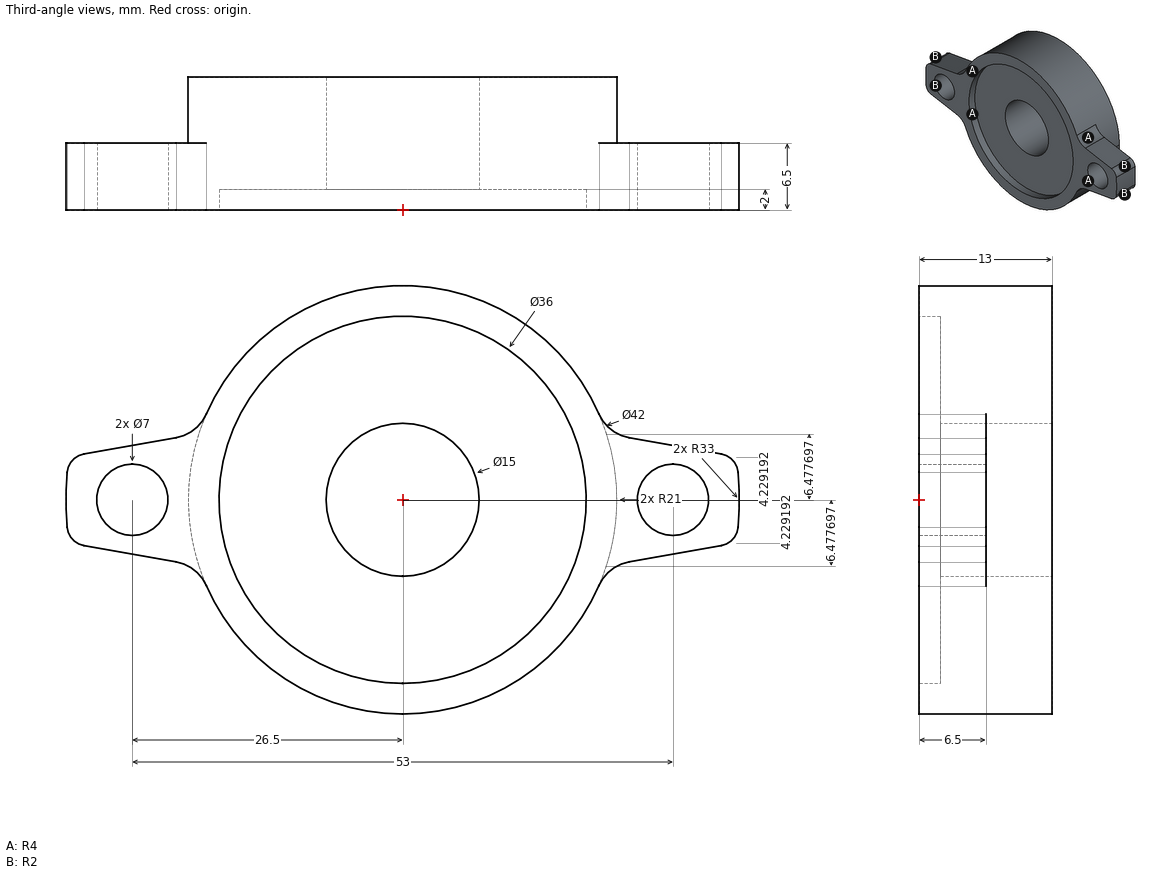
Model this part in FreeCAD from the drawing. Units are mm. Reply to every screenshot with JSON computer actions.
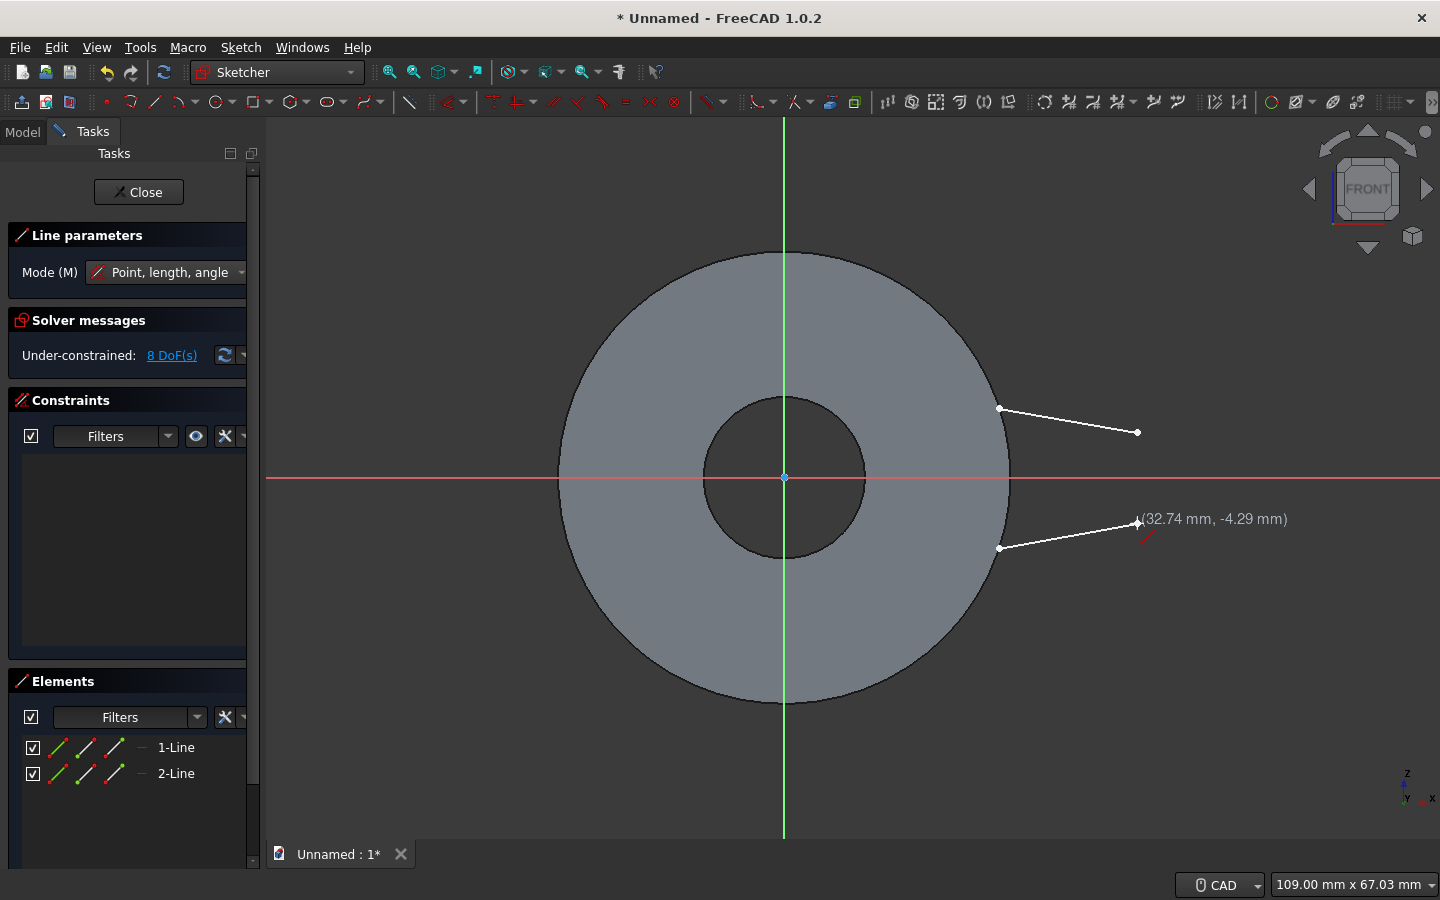
{"action": "key", "text": "g 3 a"}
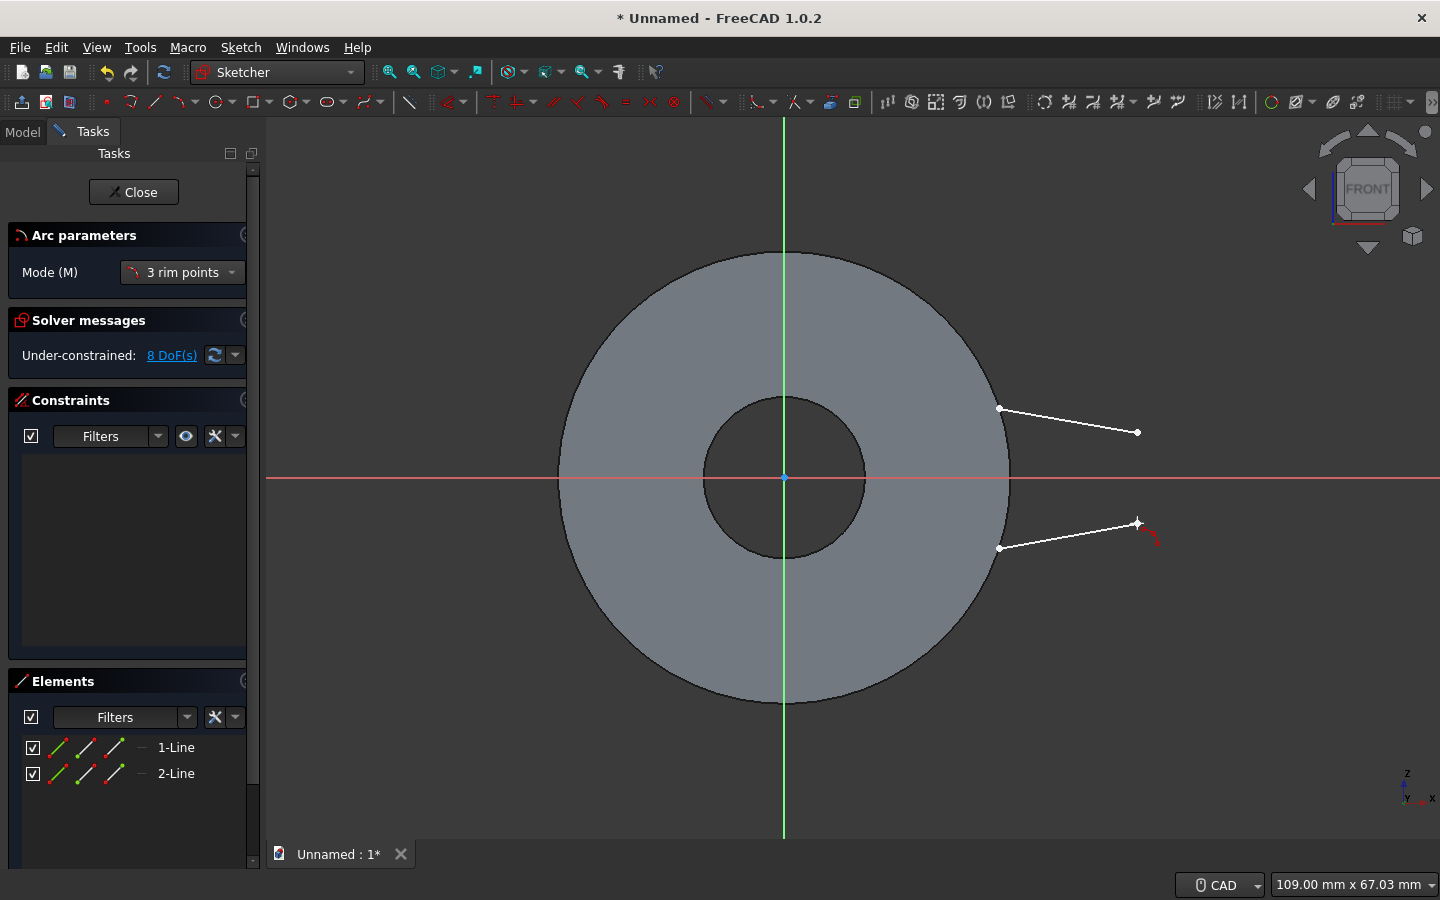
{"action": "left_click", "coordinate": [999, 409]}
{"action": "left_click", "coordinate": [999, 549]}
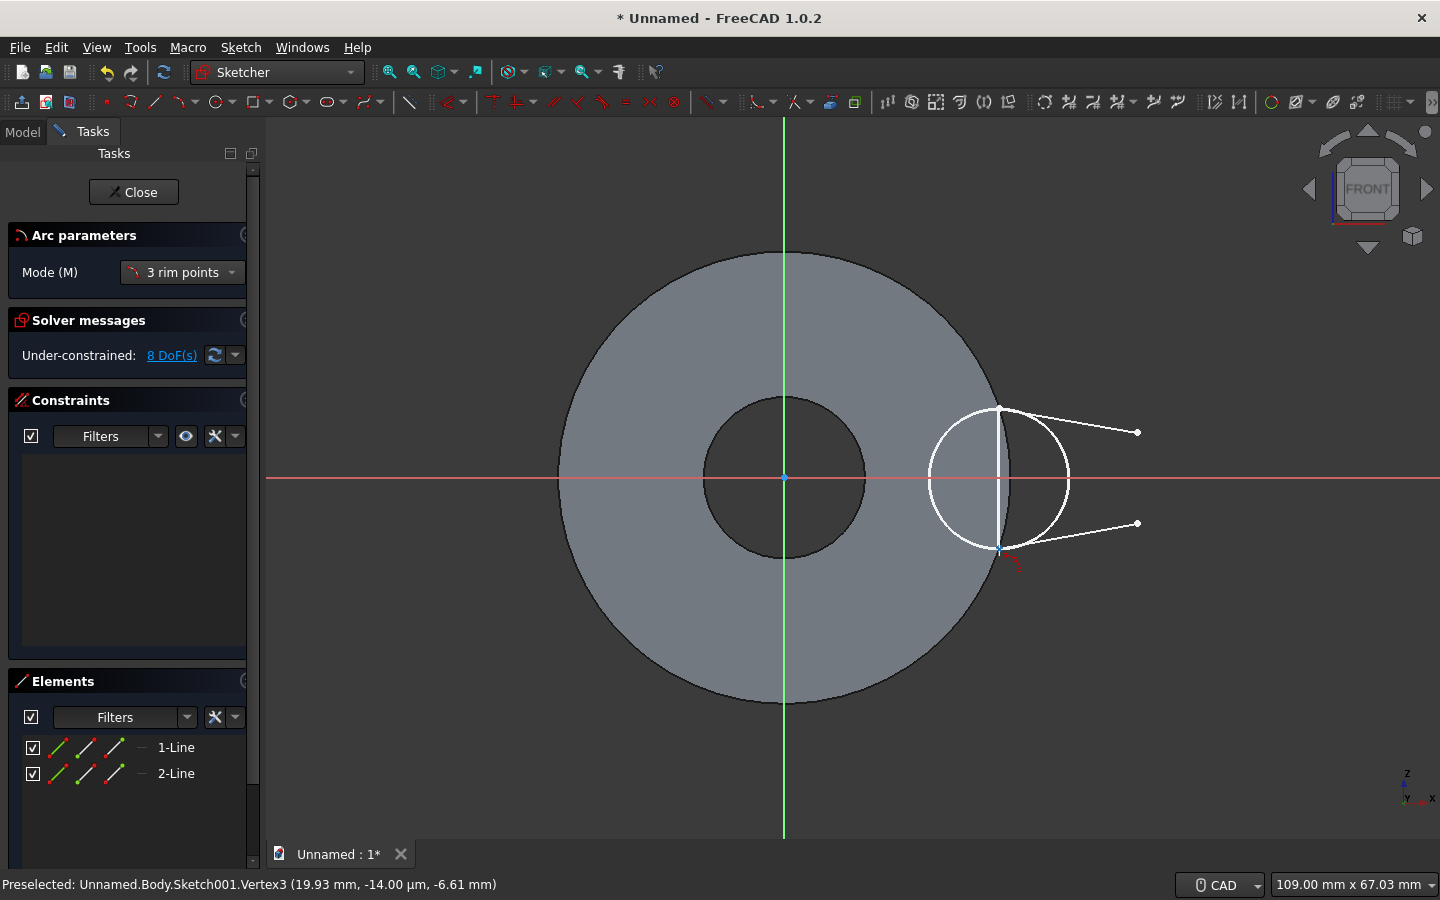
{"action": "scroll", "coordinate": [1010, 492], "scroll_direction": "up", "scroll_amount": 3}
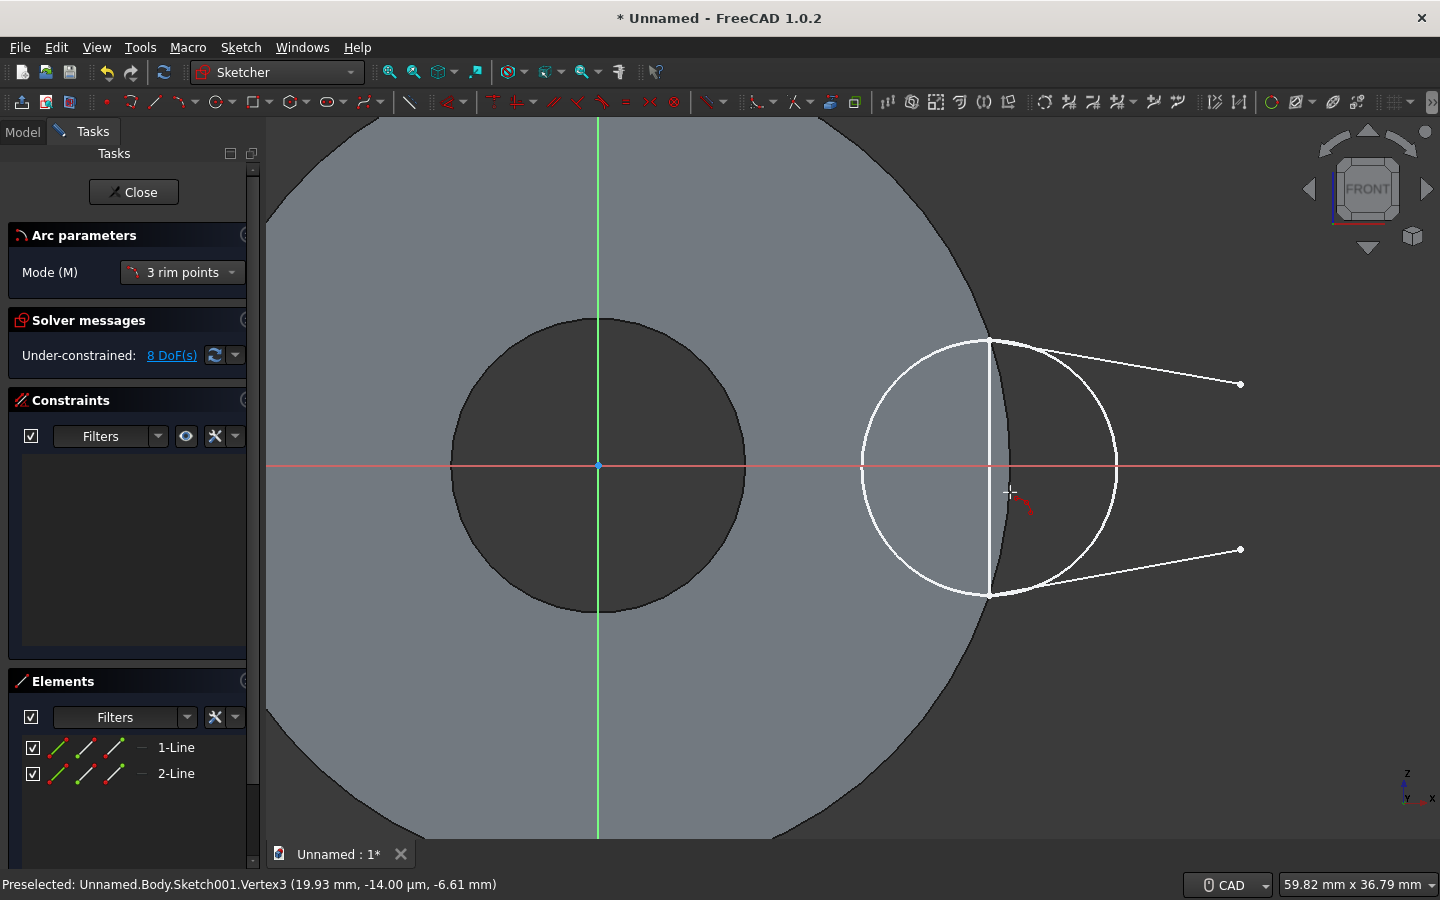
{"action": "left_click", "coordinate": [1010, 491]}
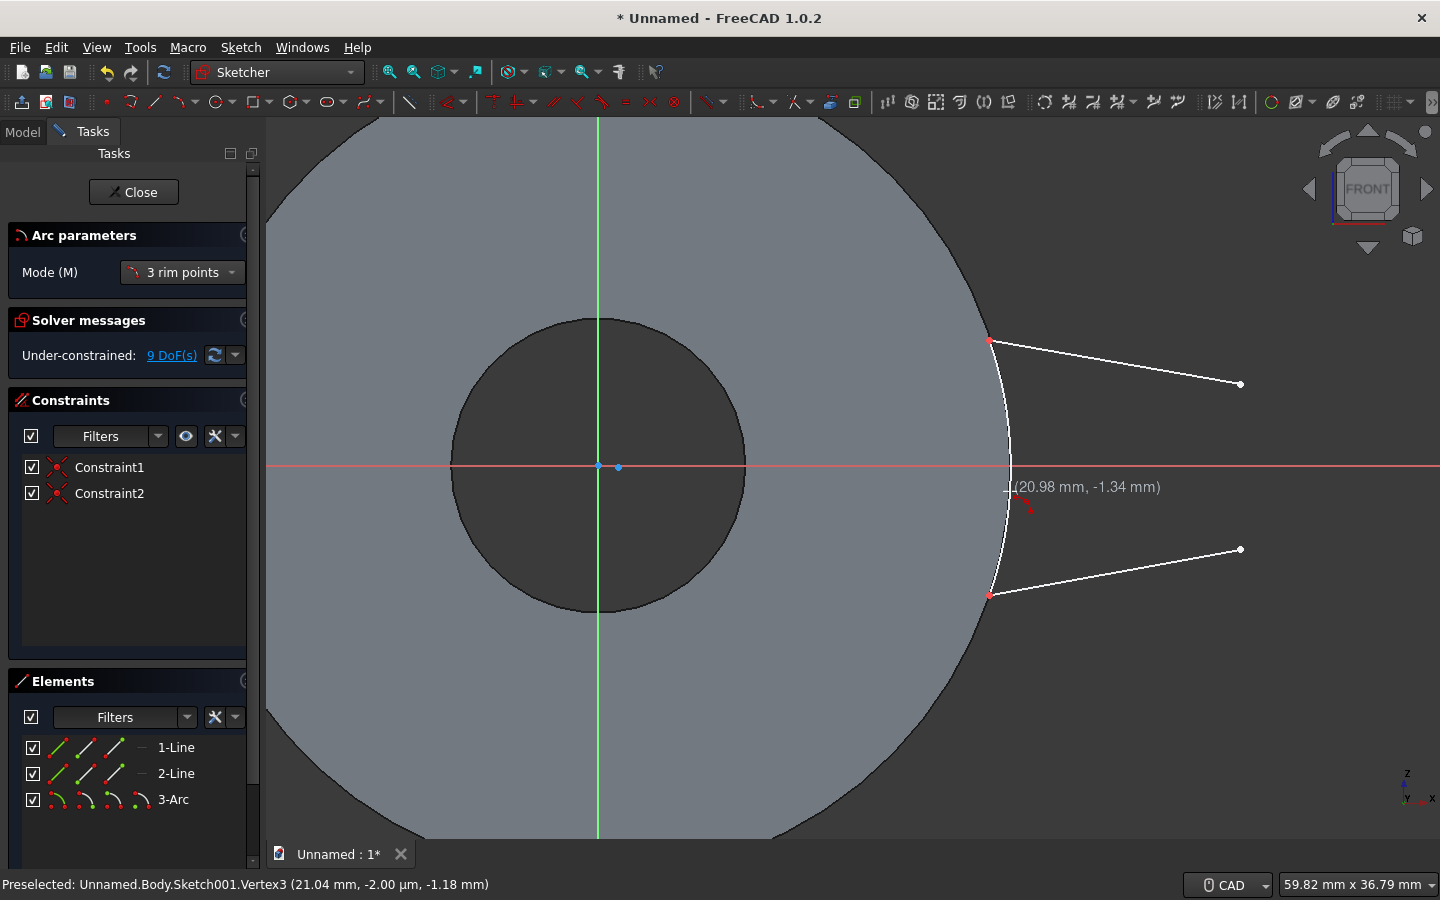
{"action": "left_click", "coordinate": [1241, 550]}
{"action": "left_click", "coordinate": [1241, 384]}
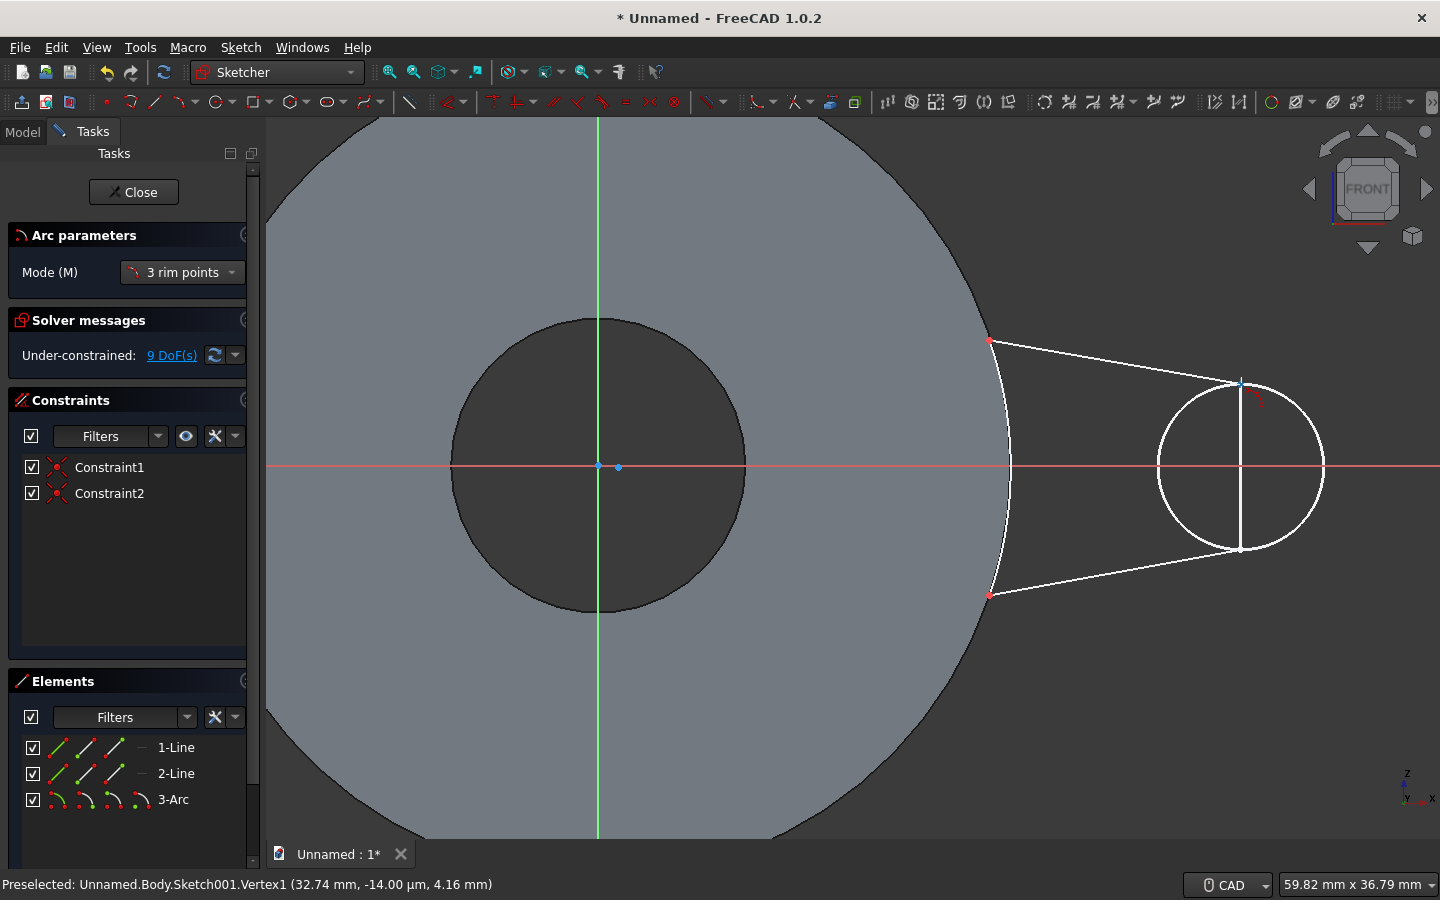
{"action": "scroll", "coordinate": [1246, 482], "scroll_direction": "up", "scroll_amount": 6}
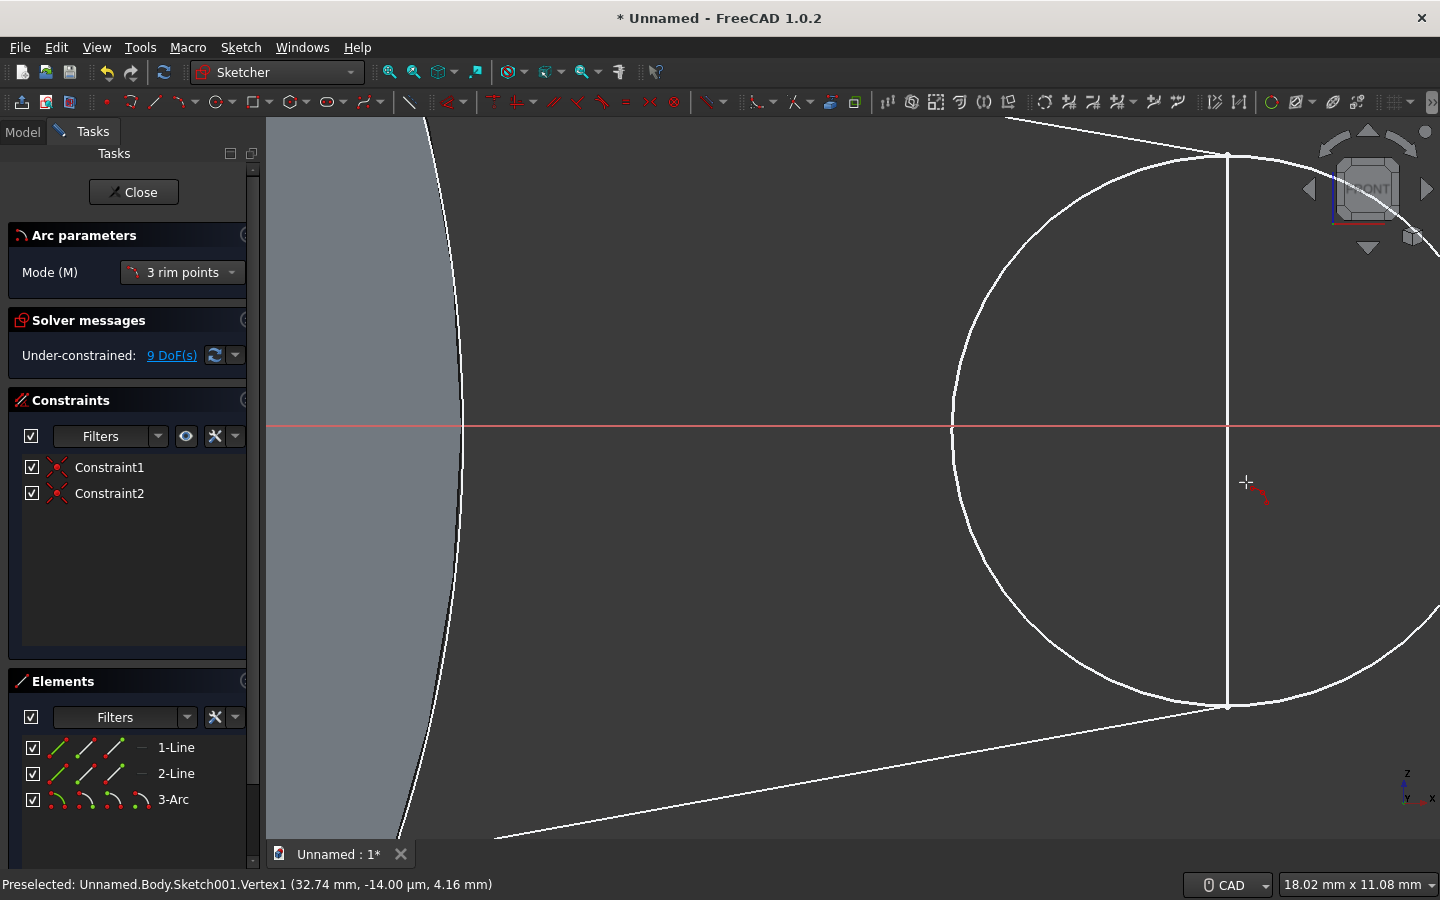
{"action": "left_click", "coordinate": [1243, 482]}